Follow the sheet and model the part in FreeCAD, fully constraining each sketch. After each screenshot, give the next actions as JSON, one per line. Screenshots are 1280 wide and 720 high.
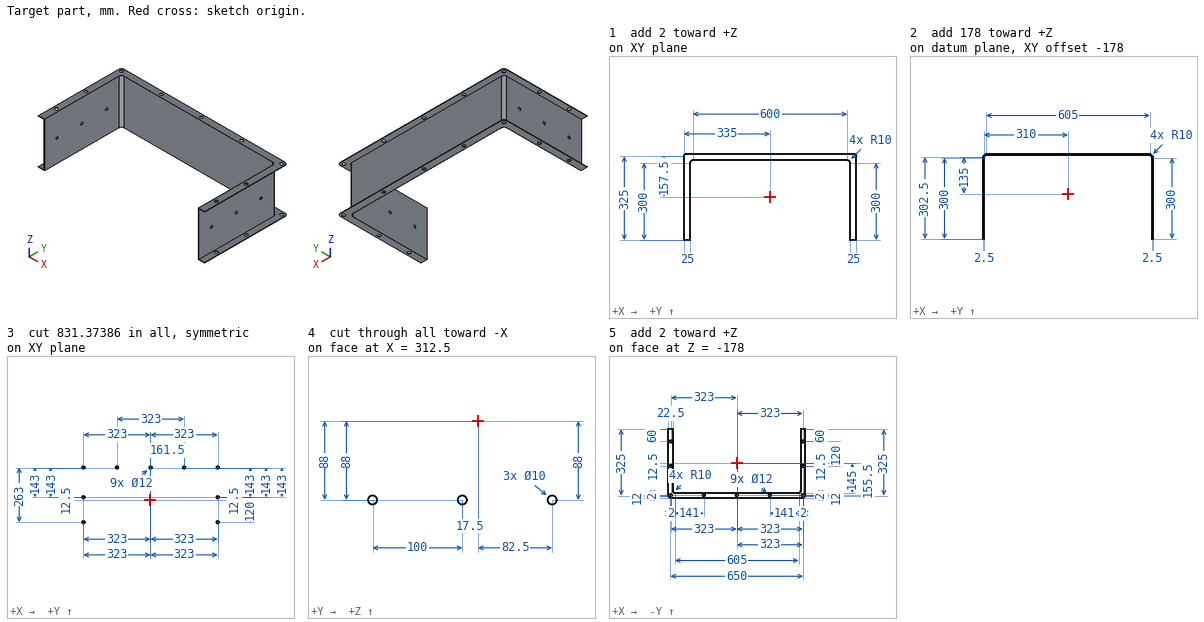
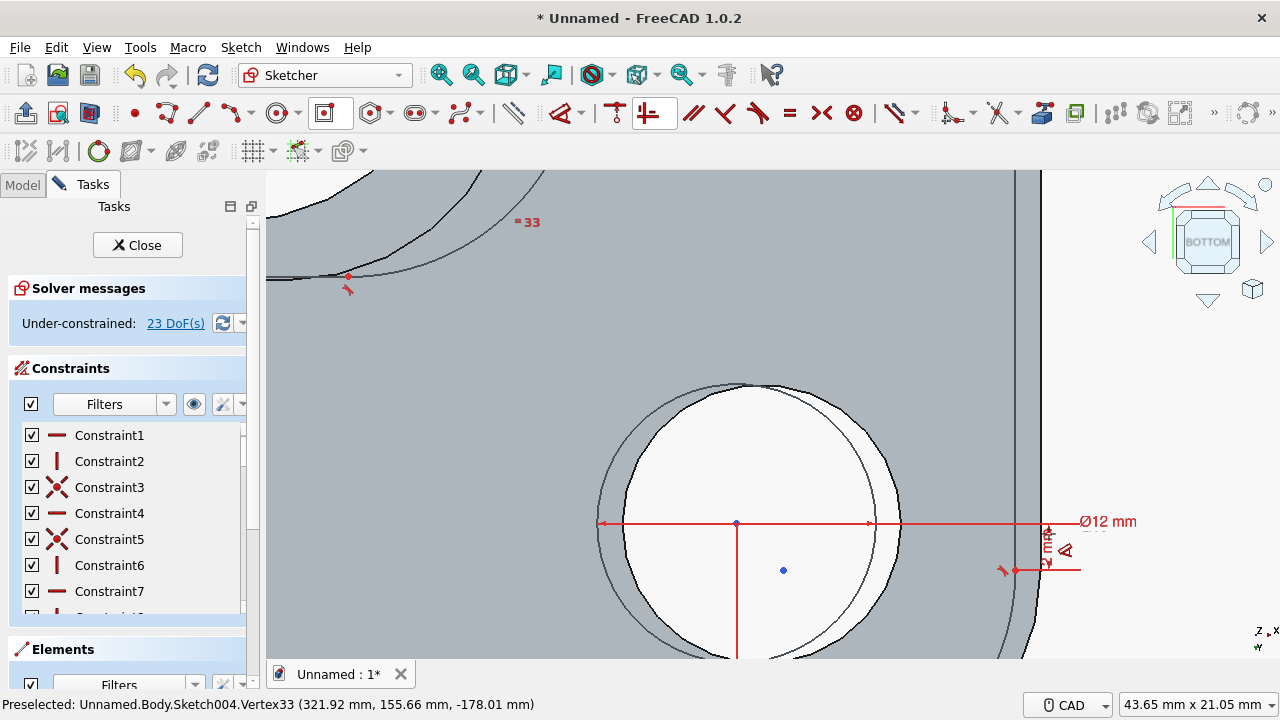
{"action": "scroll", "coordinate": [1021, 563], "scroll_direction": "down", "scroll_amount": 16}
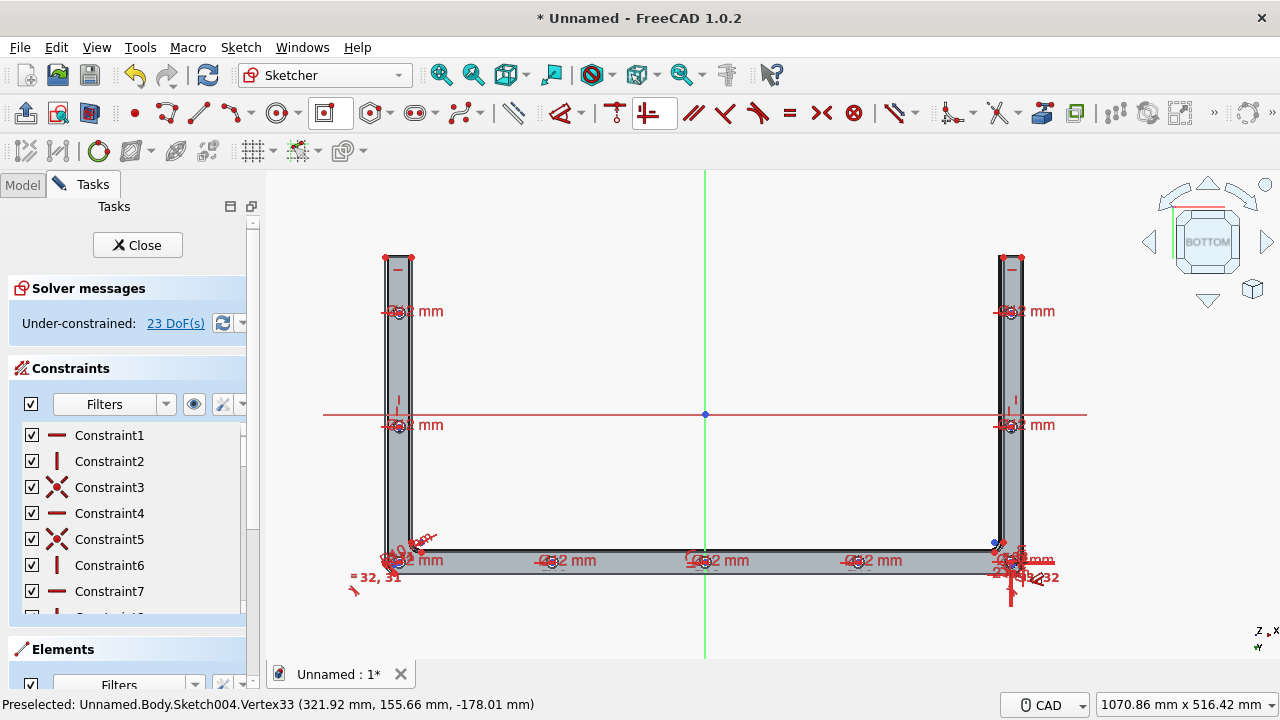
{"action": "scroll", "coordinate": [395, 574], "scroll_direction": "up", "scroll_amount": 16}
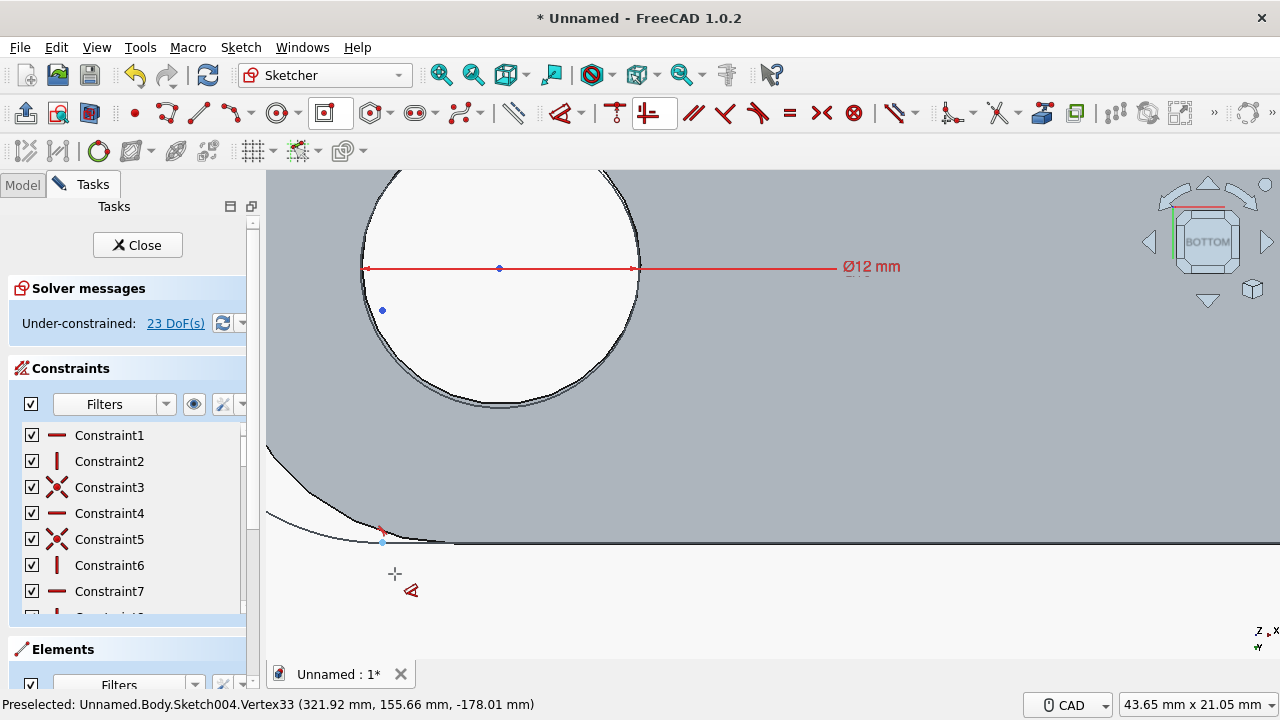
{"action": "left_click", "coordinate": [382, 543]}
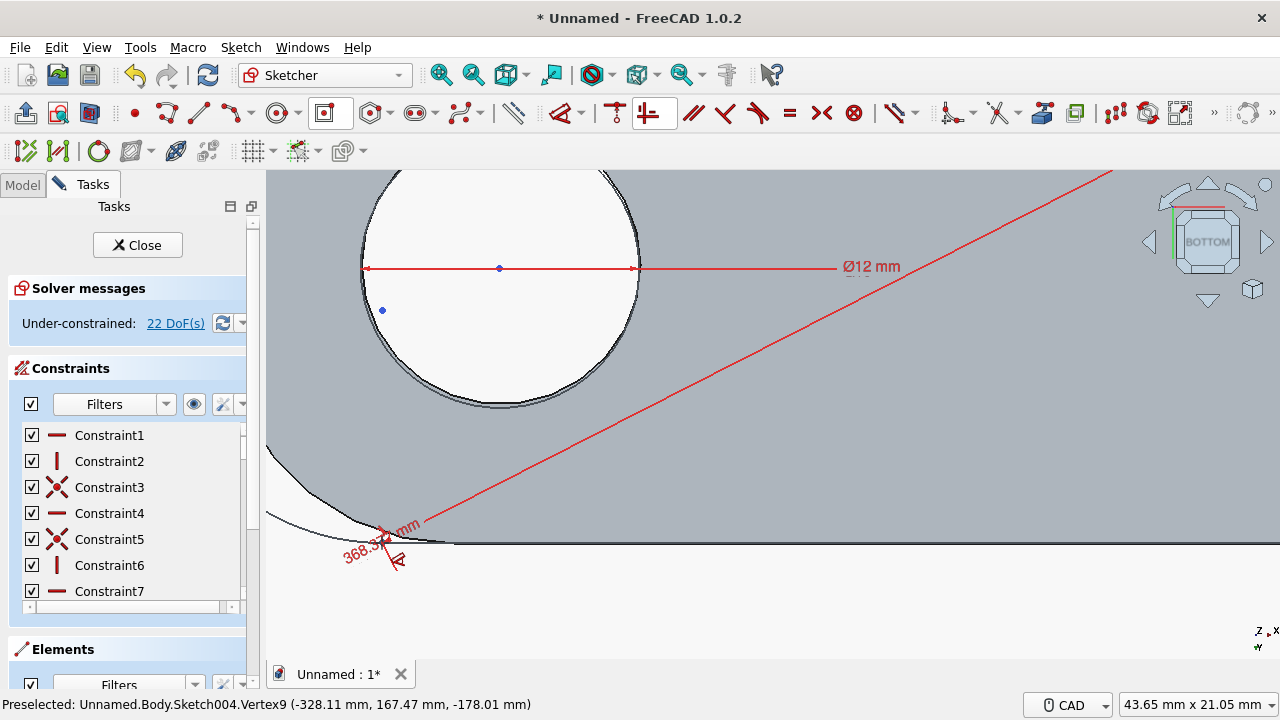
{"action": "left_click", "coordinate": [500, 269]}
{"action": "left_click", "coordinate": [441, 577]}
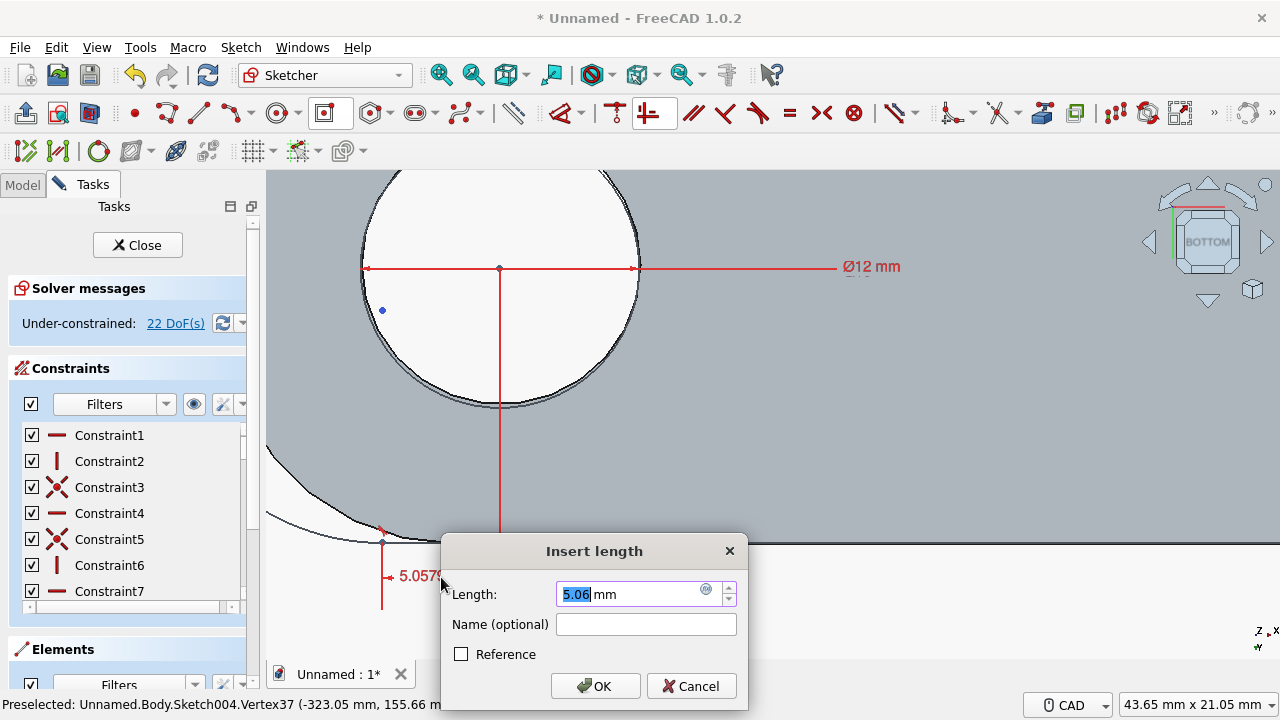
{"action": "type", "text": "2"}
{"action": "key", "text": "Return"}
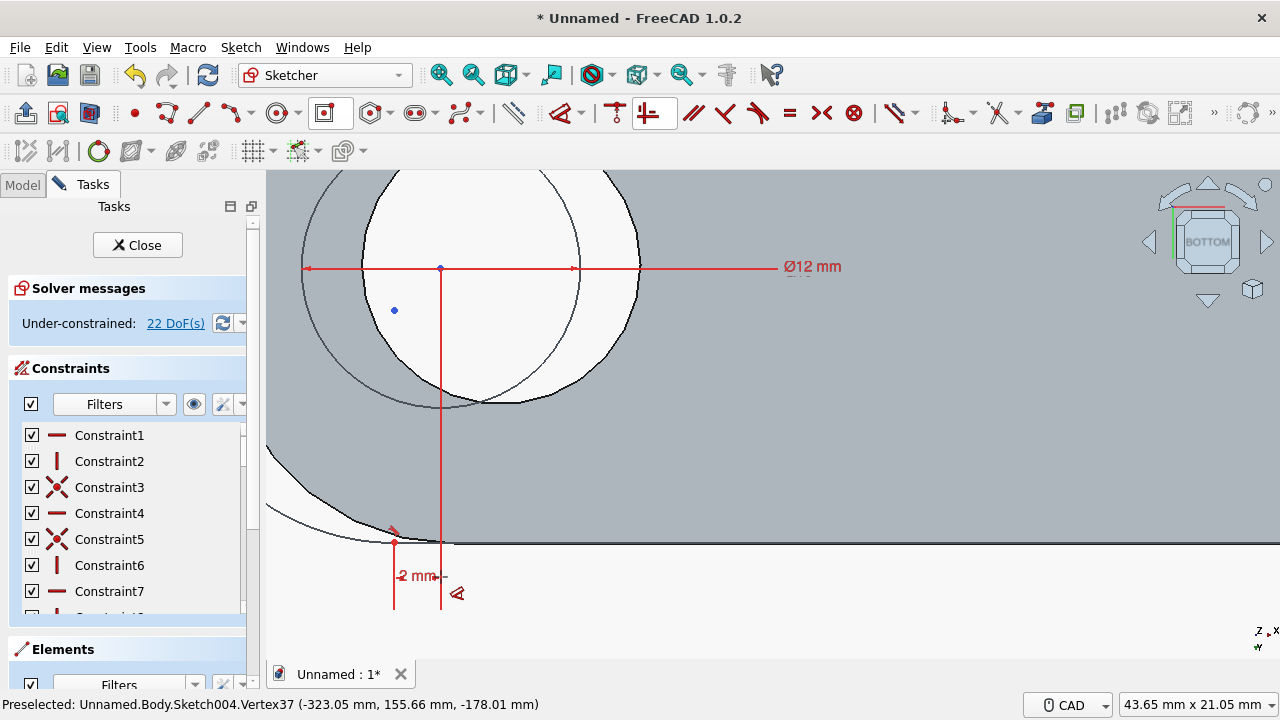
{"action": "scroll", "coordinate": [394, 574], "scroll_direction": "down", "scroll_amount": 16}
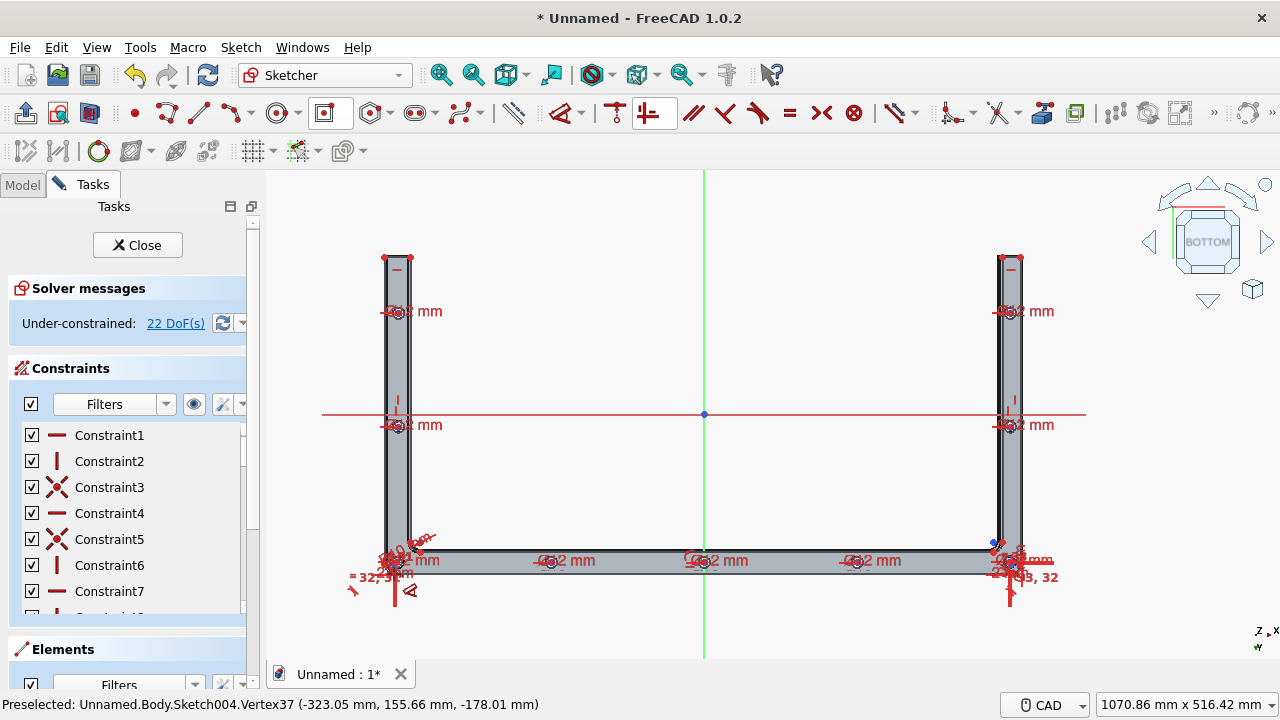
{"action": "scroll", "coordinate": [385, 564], "scroll_direction": "up", "scroll_amount": 16}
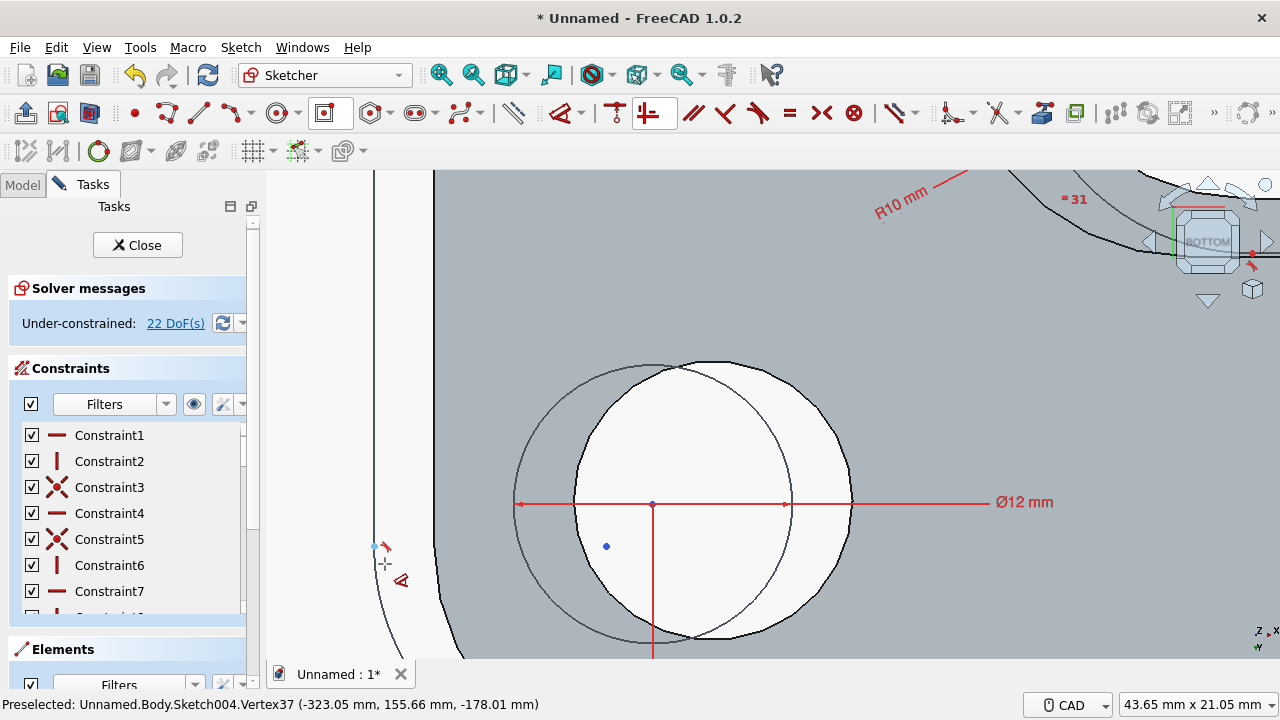
{"action": "left_click", "coordinate": [374, 546]}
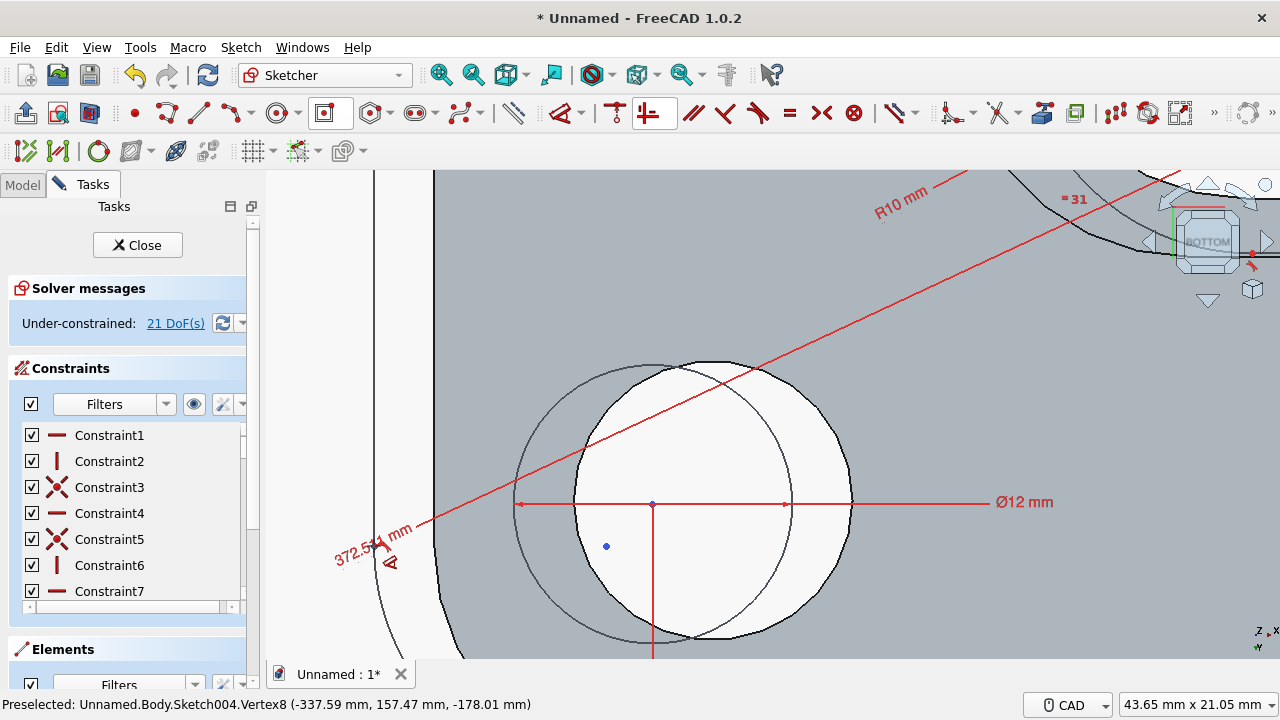
{"action": "left_click", "coordinate": [653, 504]}
{"action": "left_click", "coordinate": [340, 525]}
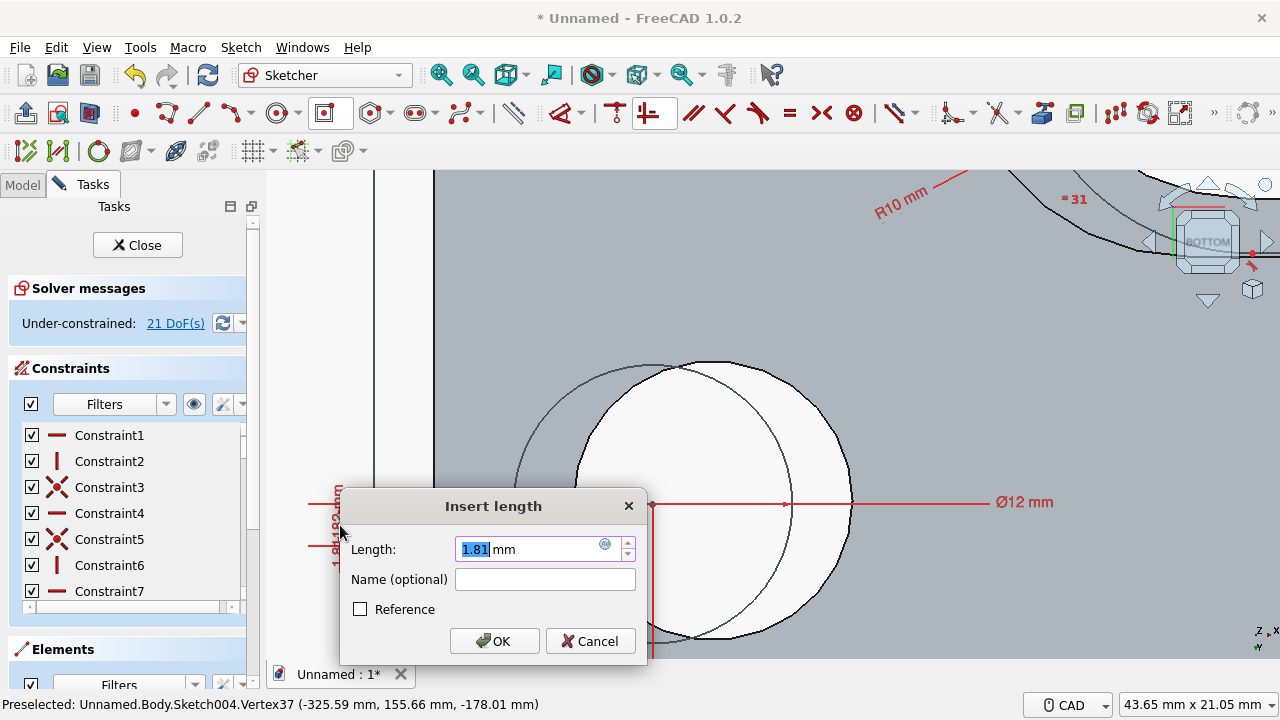
{"action": "type", "text": "2"}
{"action": "key", "text": "Return"}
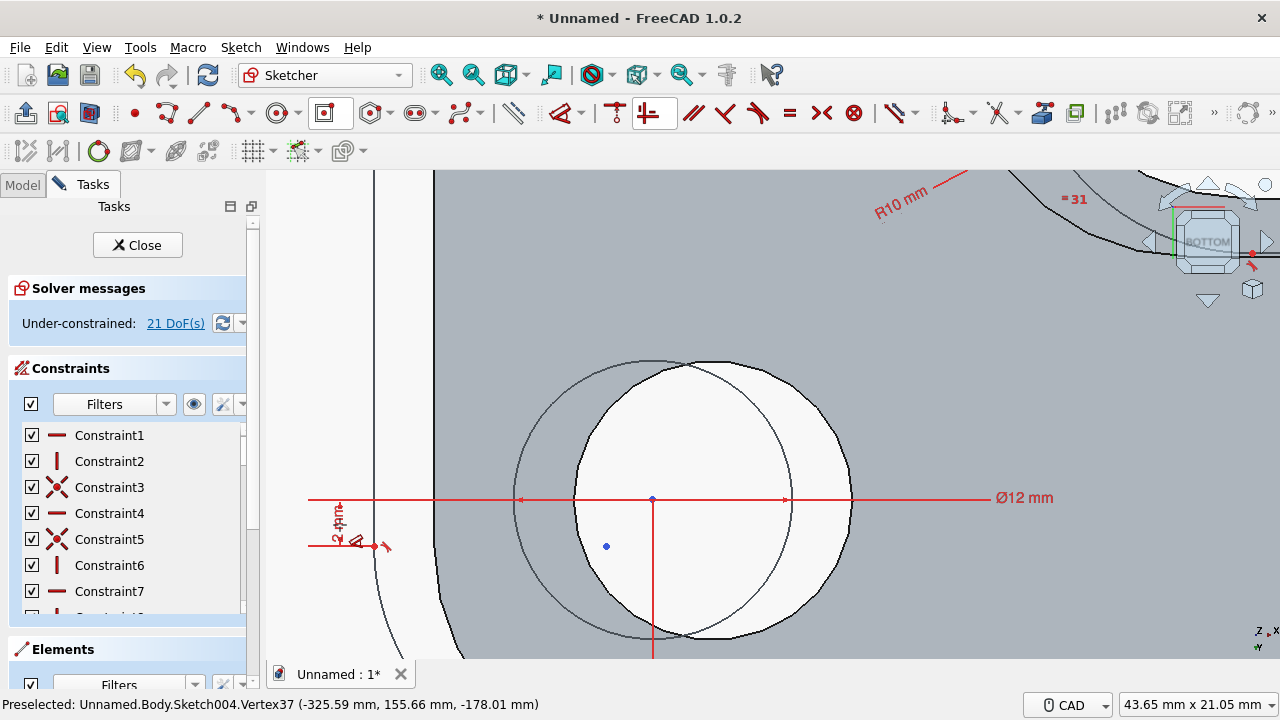
{"action": "scroll", "coordinate": [385, 564], "scroll_direction": "down", "scroll_amount": 16}